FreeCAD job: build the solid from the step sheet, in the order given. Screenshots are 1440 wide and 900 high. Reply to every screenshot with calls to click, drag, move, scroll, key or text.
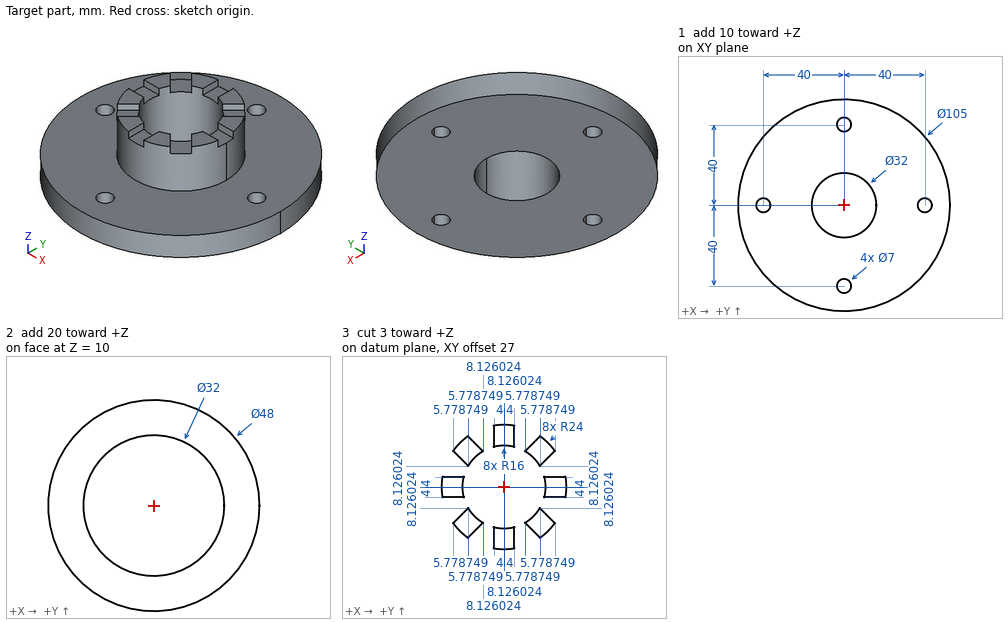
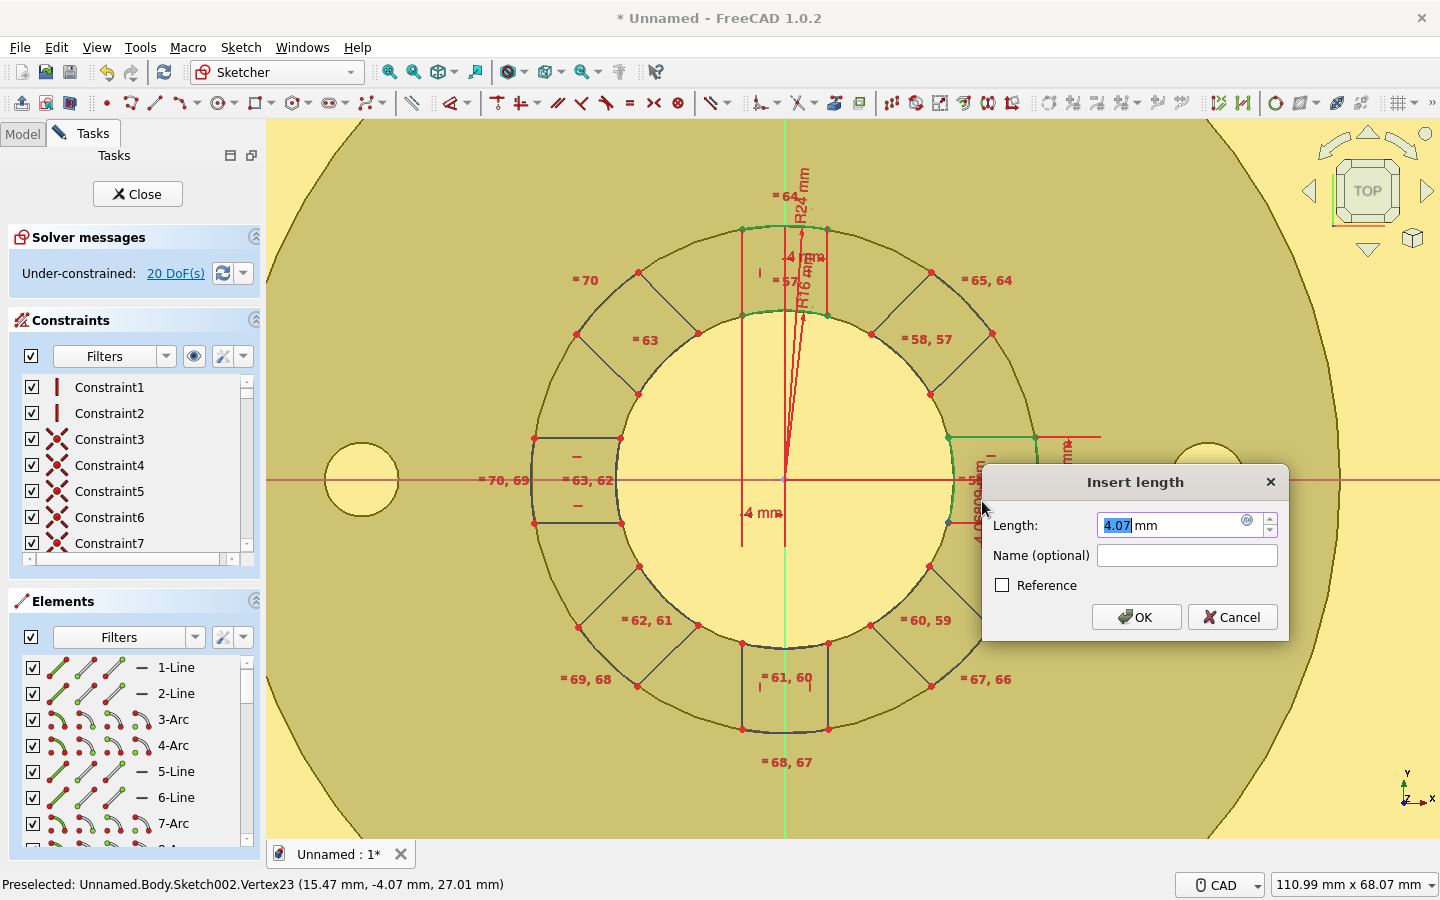
text(4)
key(Return)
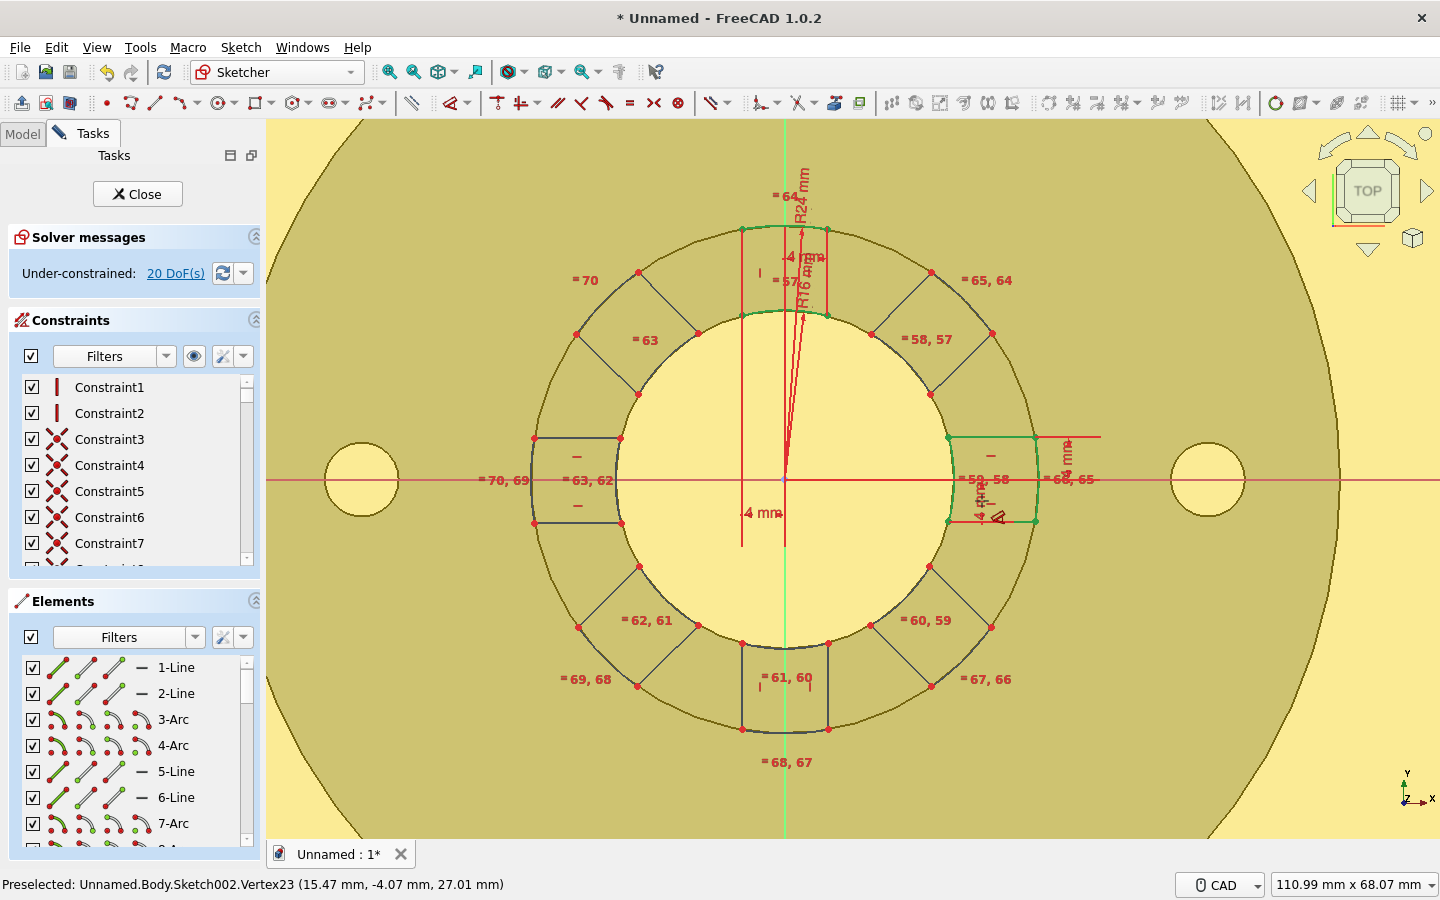
click(828, 730)
click(806, 764)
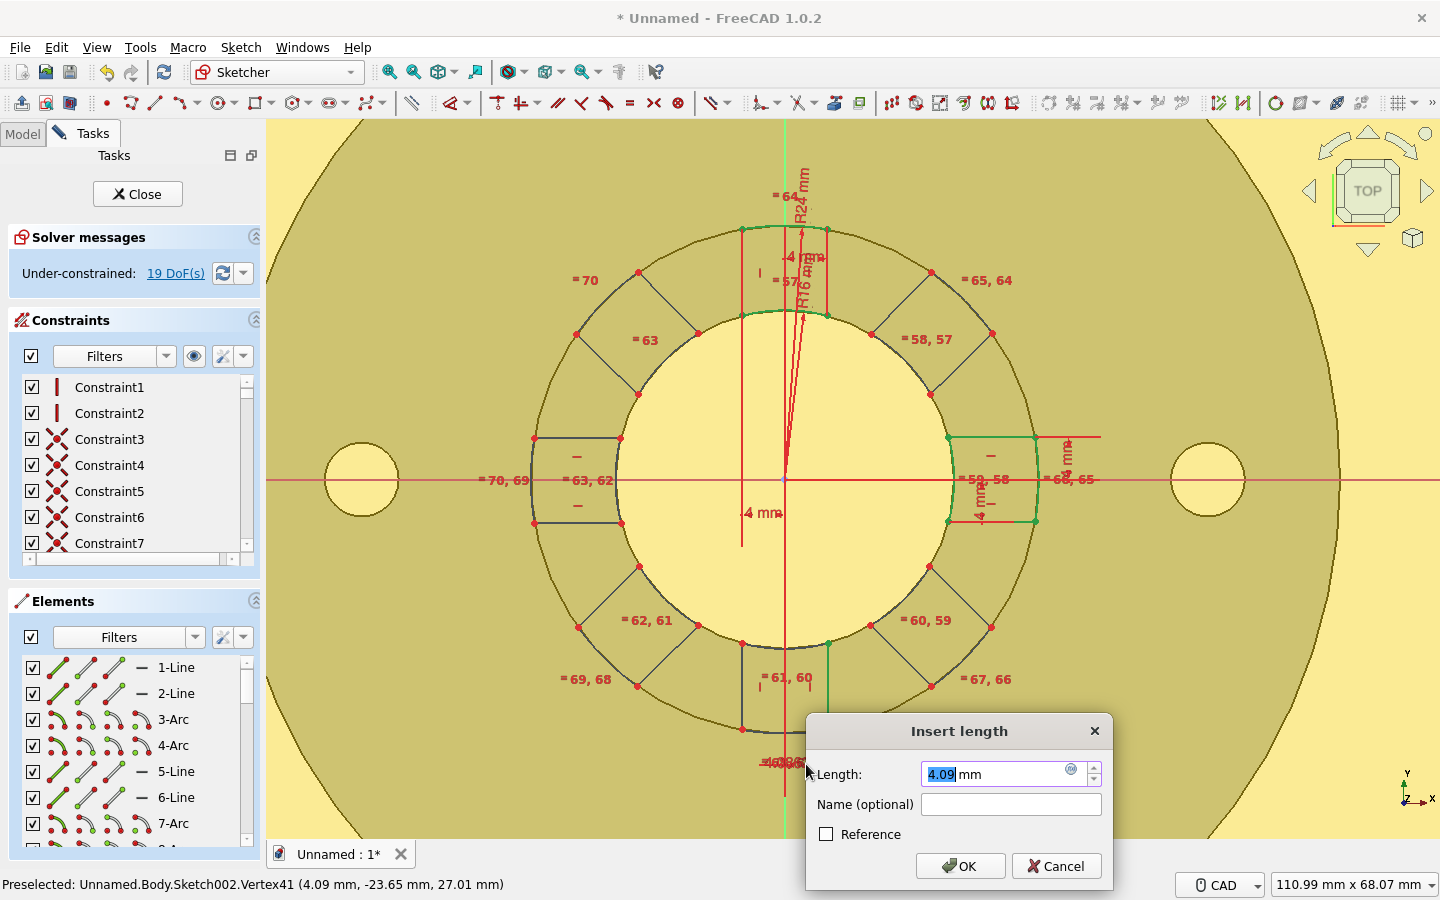
text(4)
key(Return)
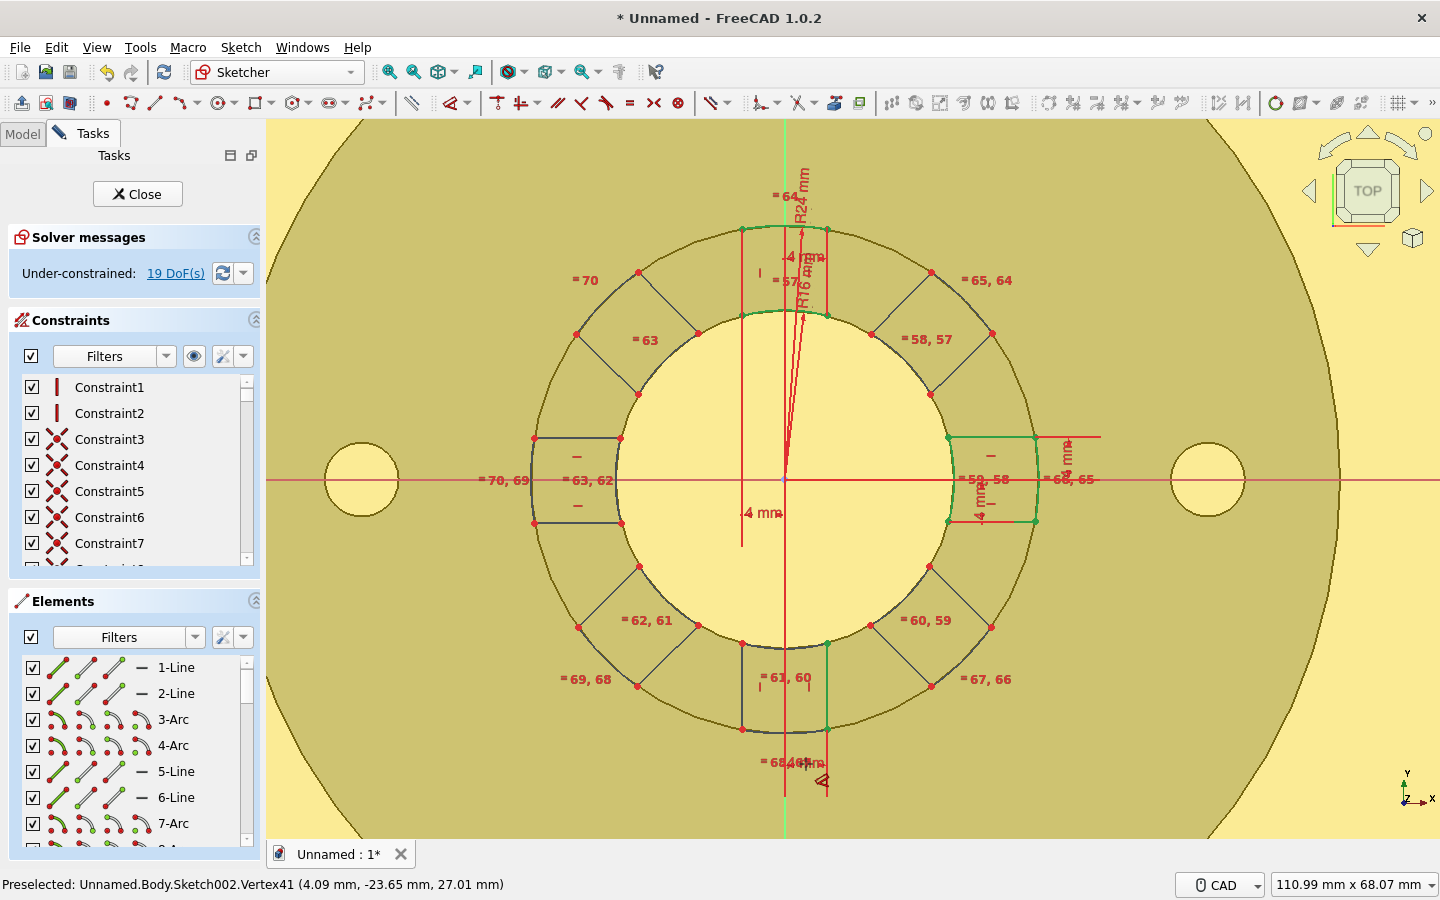
click(742, 643)
click(763, 677)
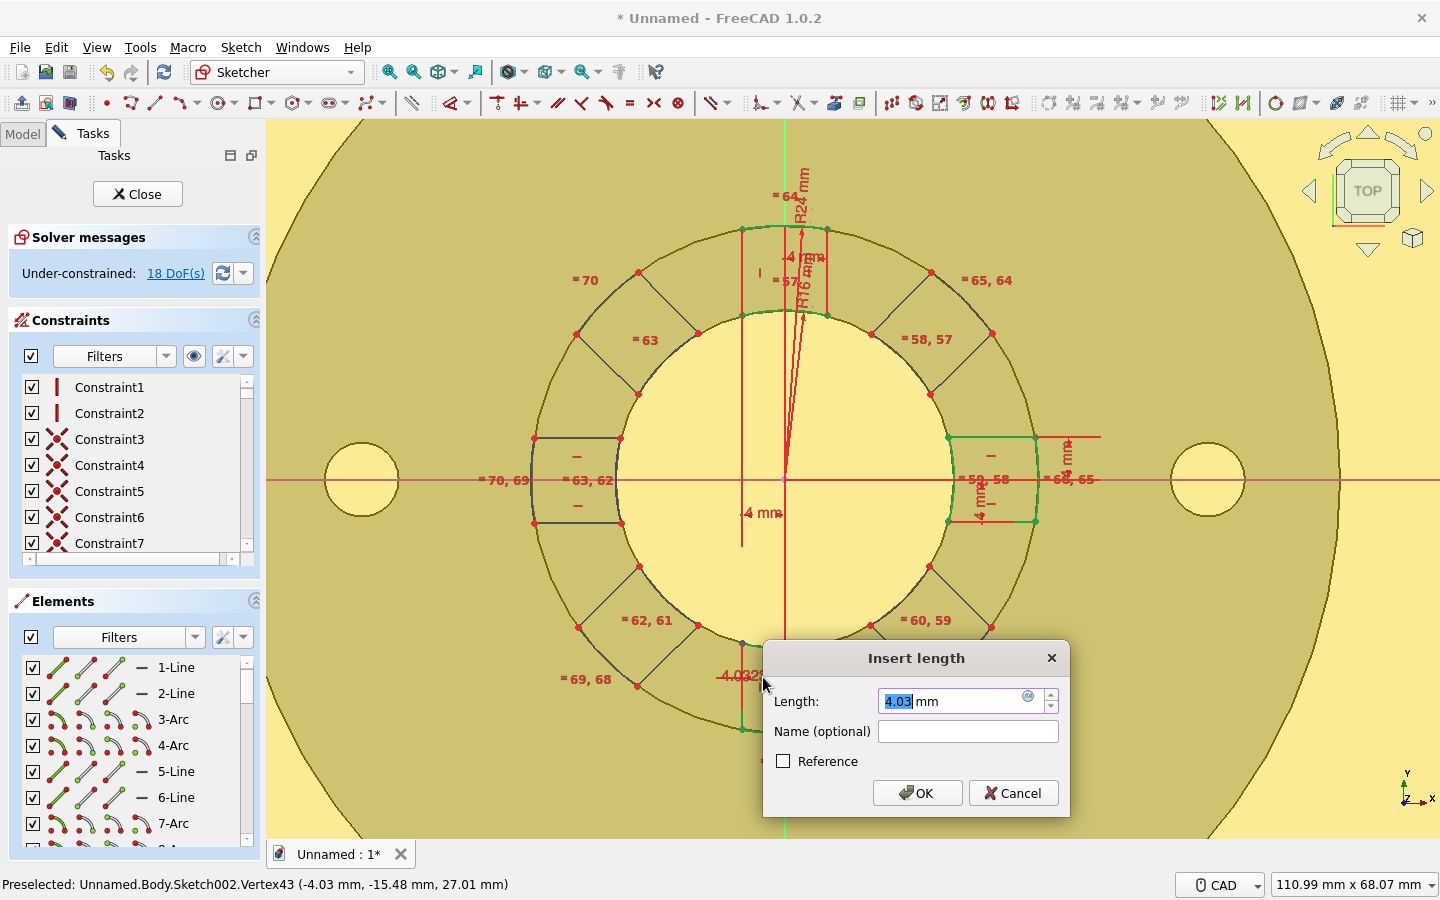
text(4)
key(Return)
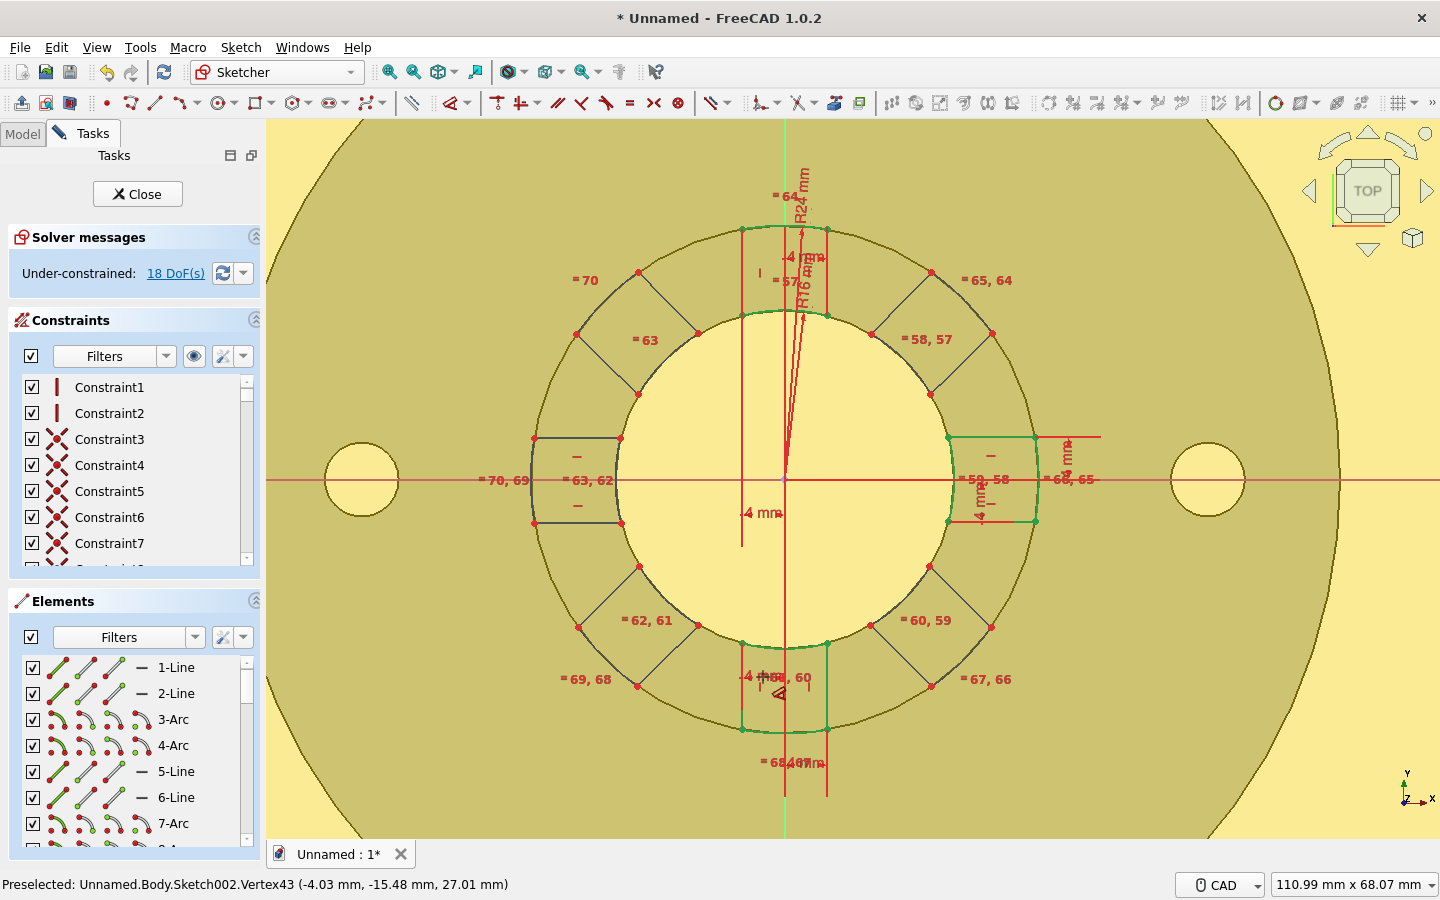
click(535, 523)
click(501, 501)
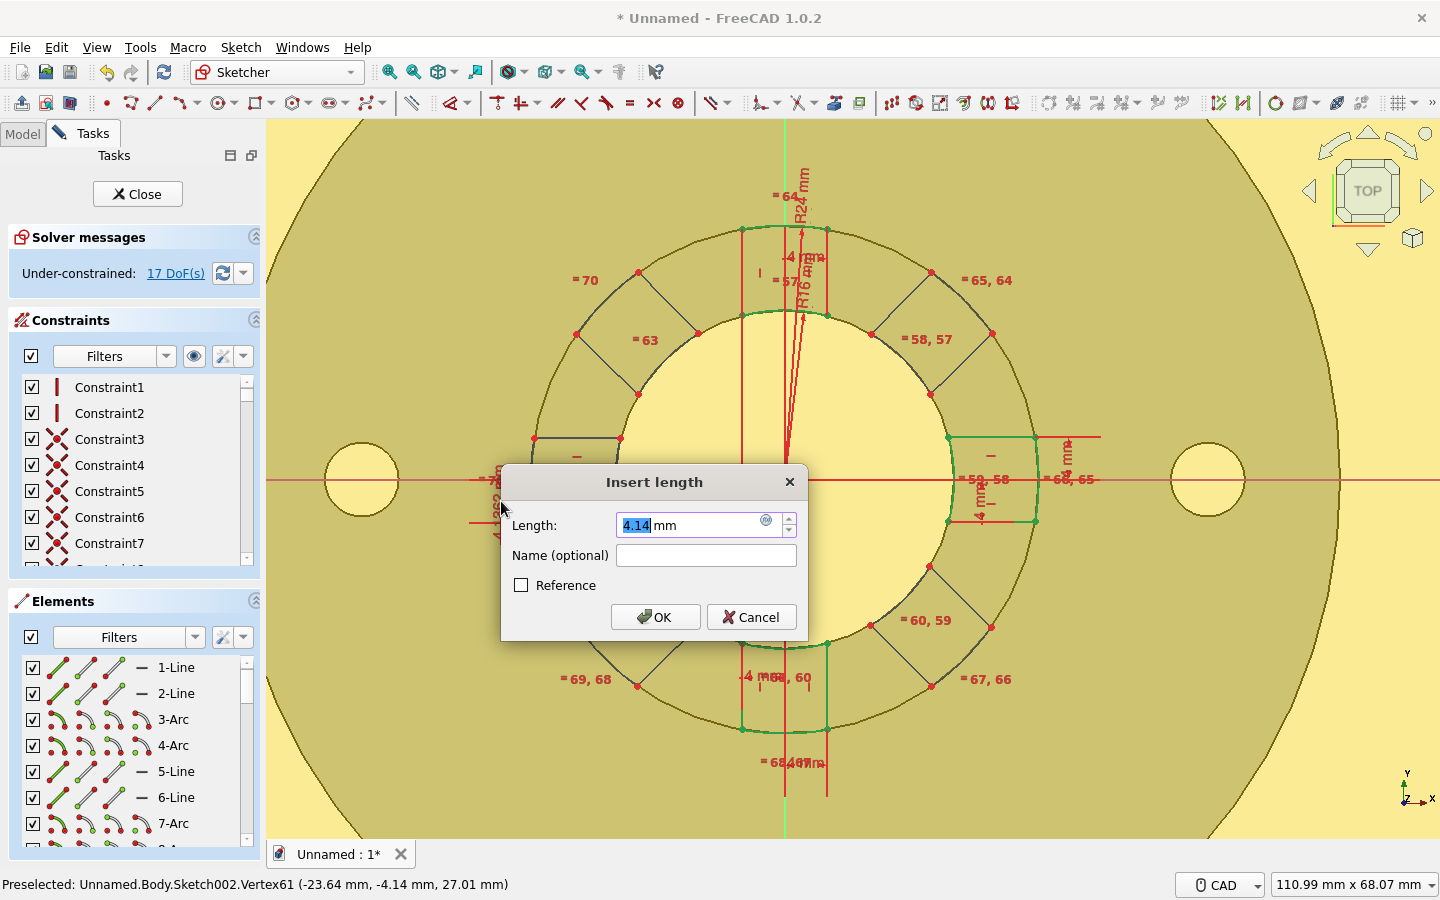
text(4)
key(Return)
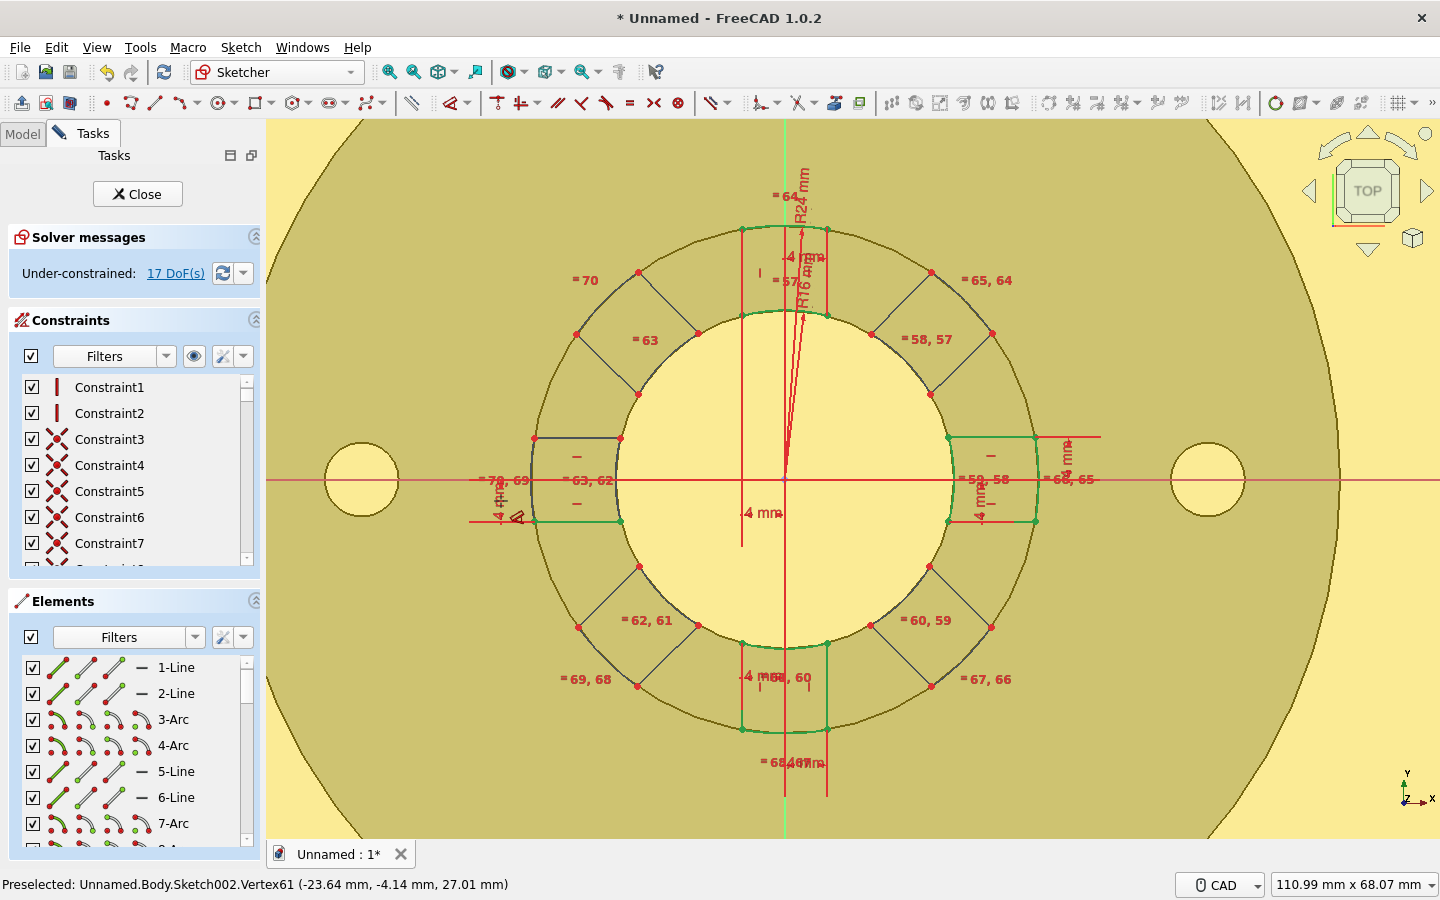
click(621, 438)
click(587, 459)